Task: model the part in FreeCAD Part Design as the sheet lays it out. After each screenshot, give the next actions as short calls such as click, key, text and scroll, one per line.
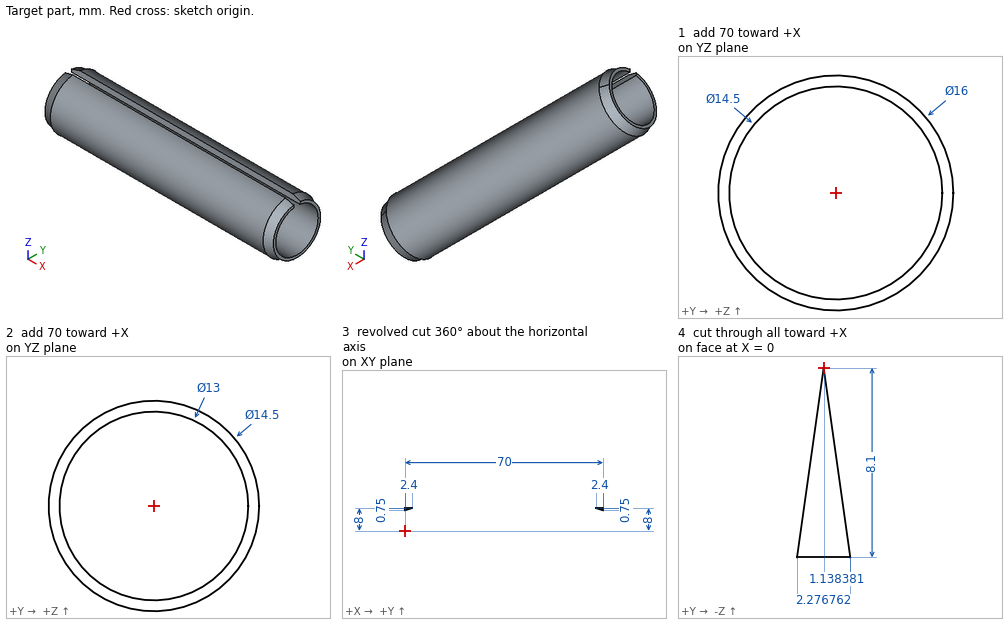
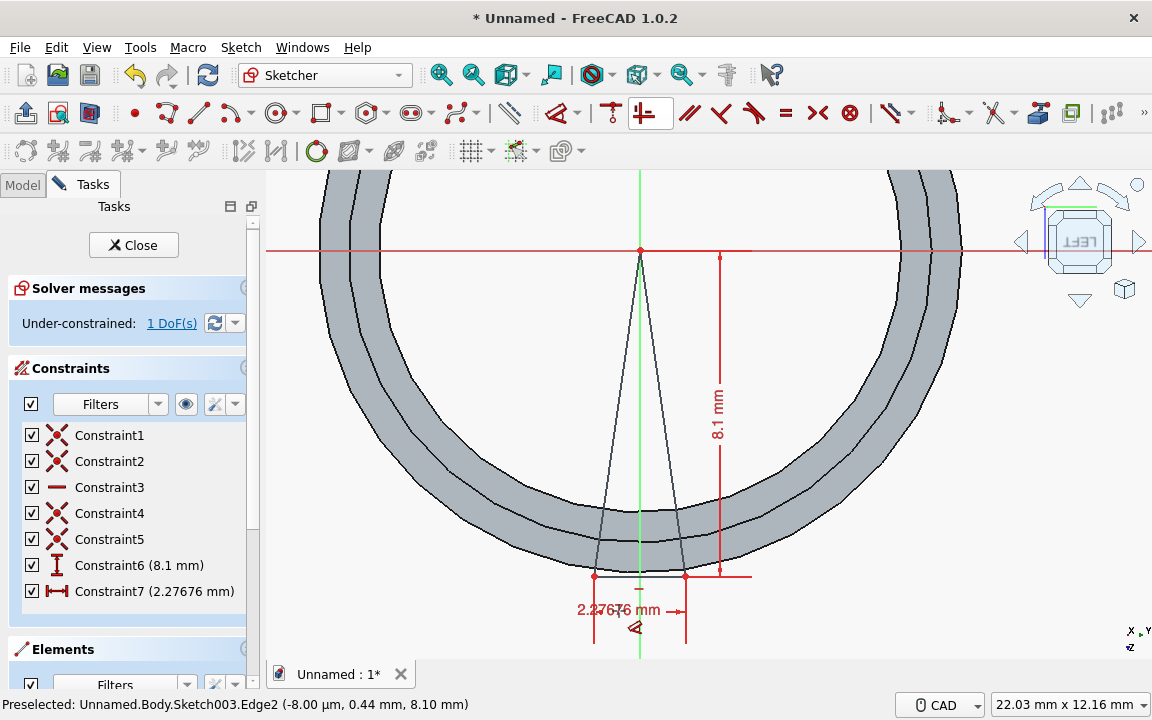
click(686, 577)
click(663, 217)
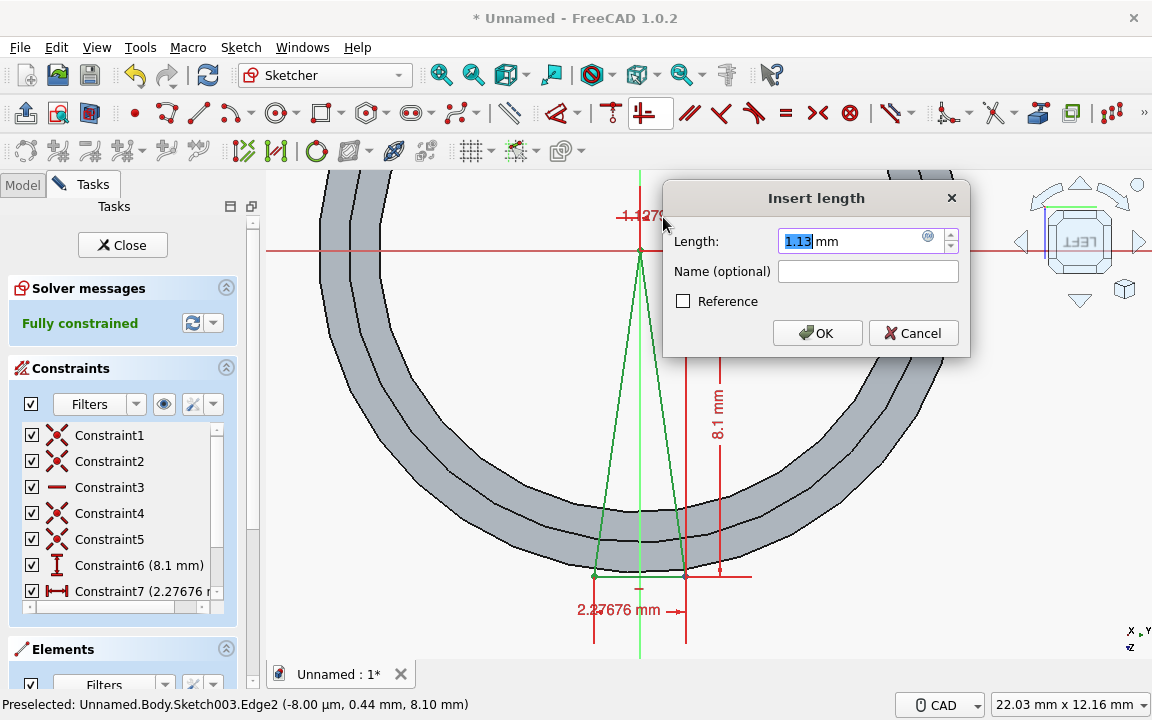
text(1.138381)
key(Return)
key(Escape)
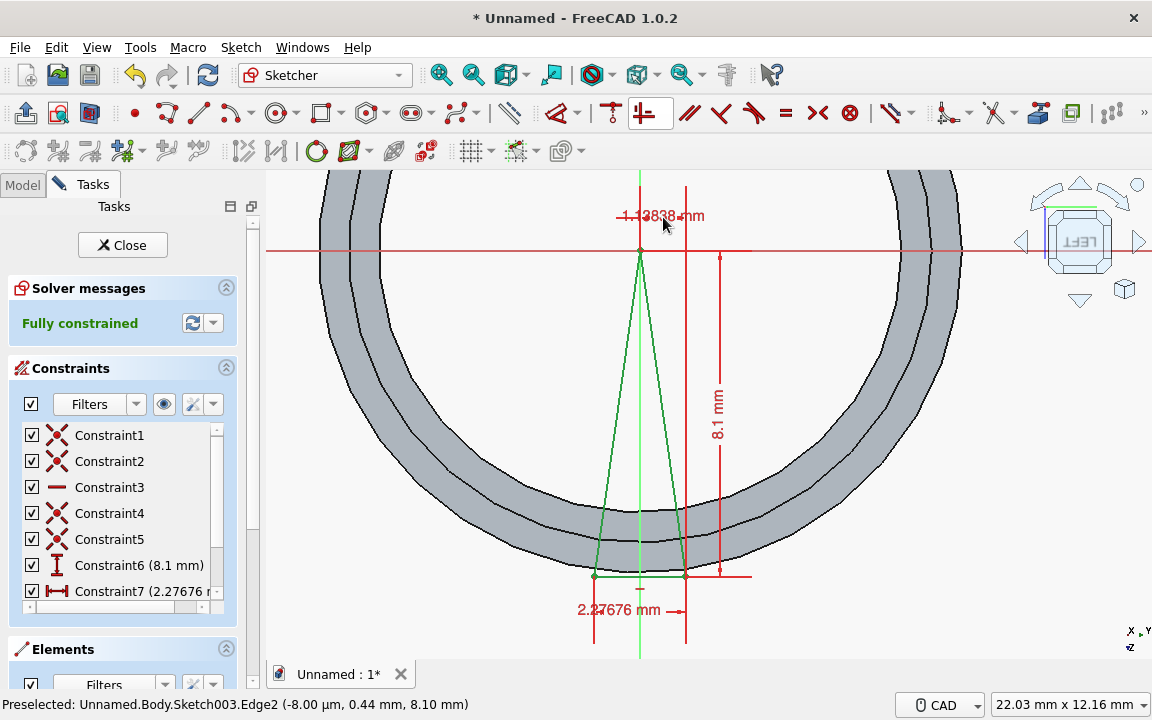
click(123, 245)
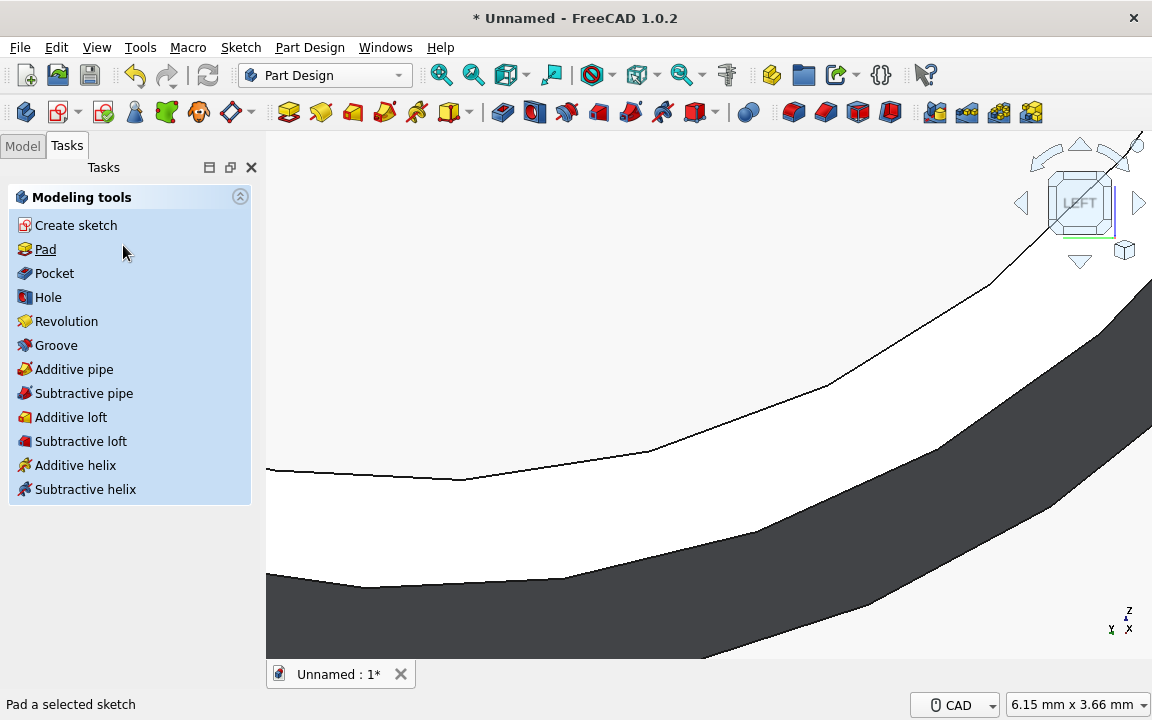
click(504, 112)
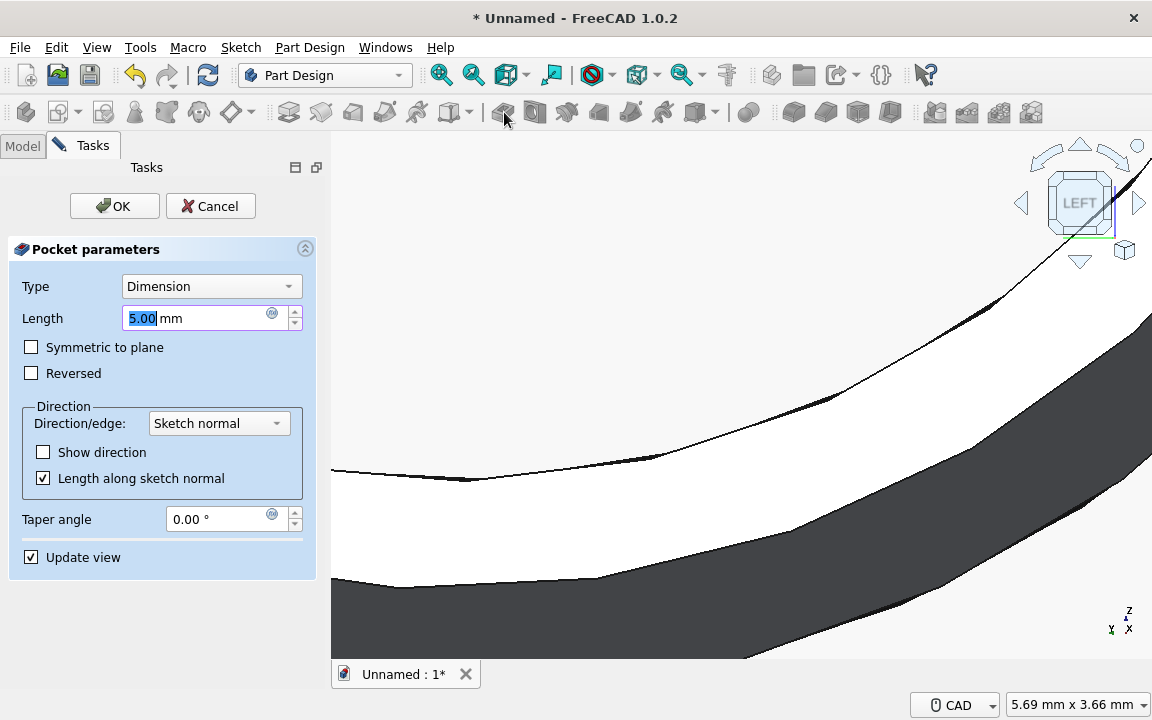
click(212, 286)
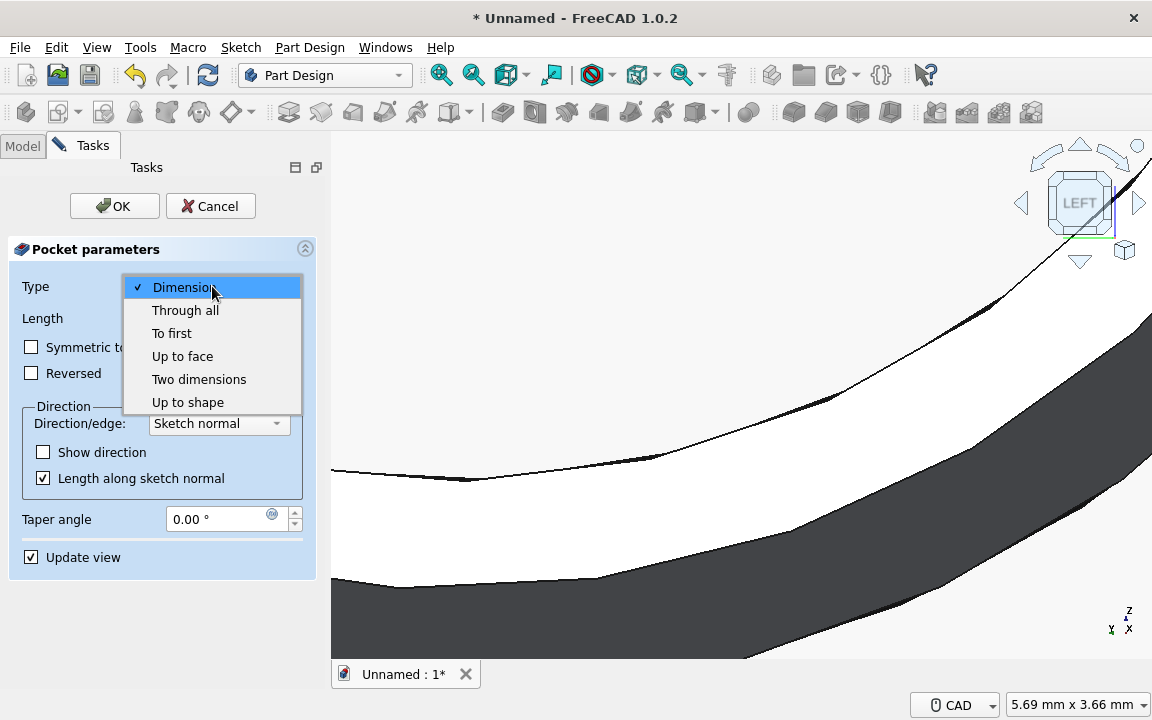
click(212, 310)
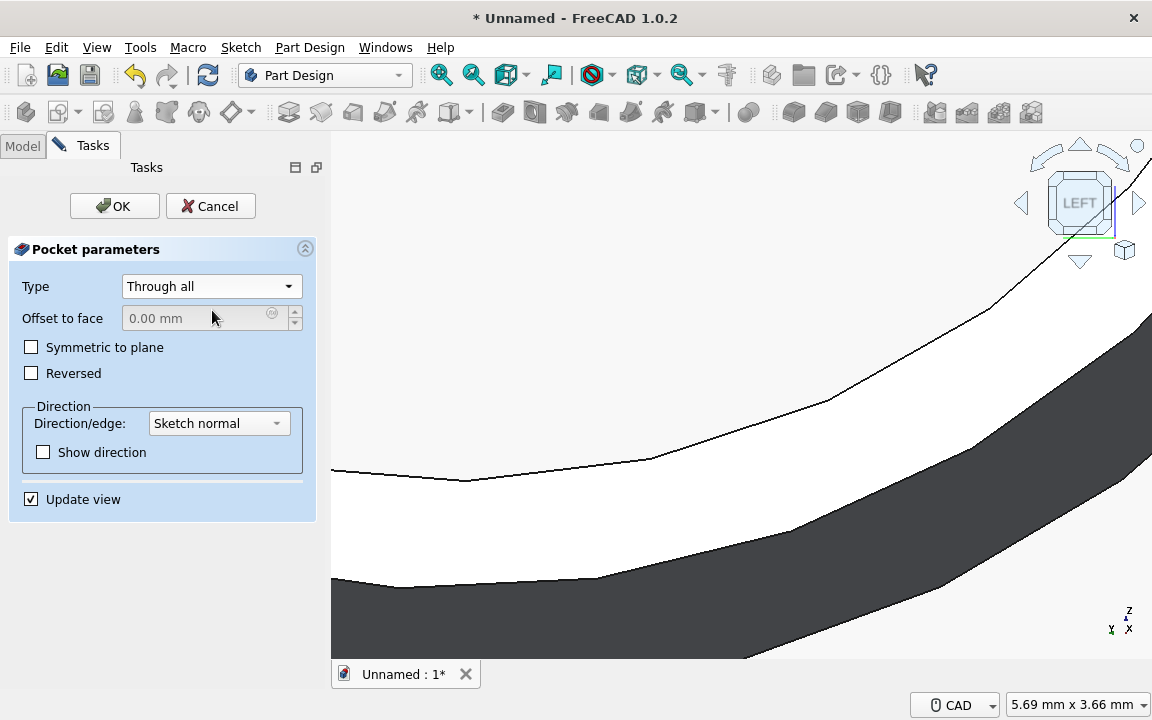
click(115, 206)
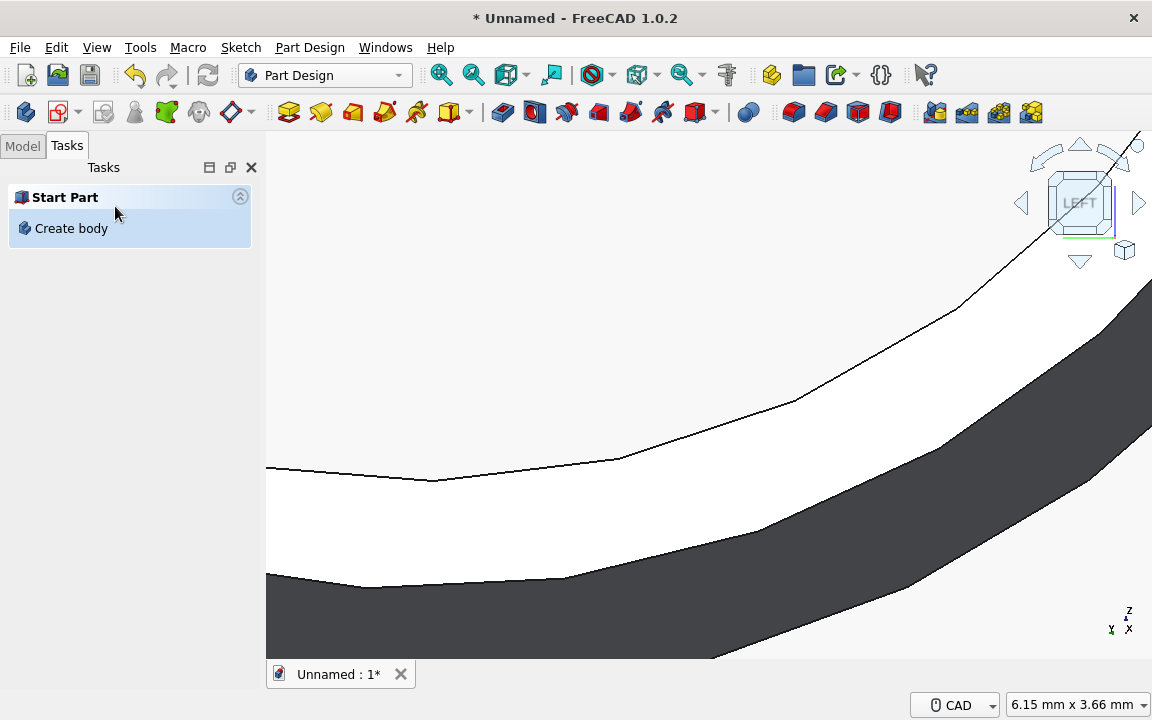
key(0)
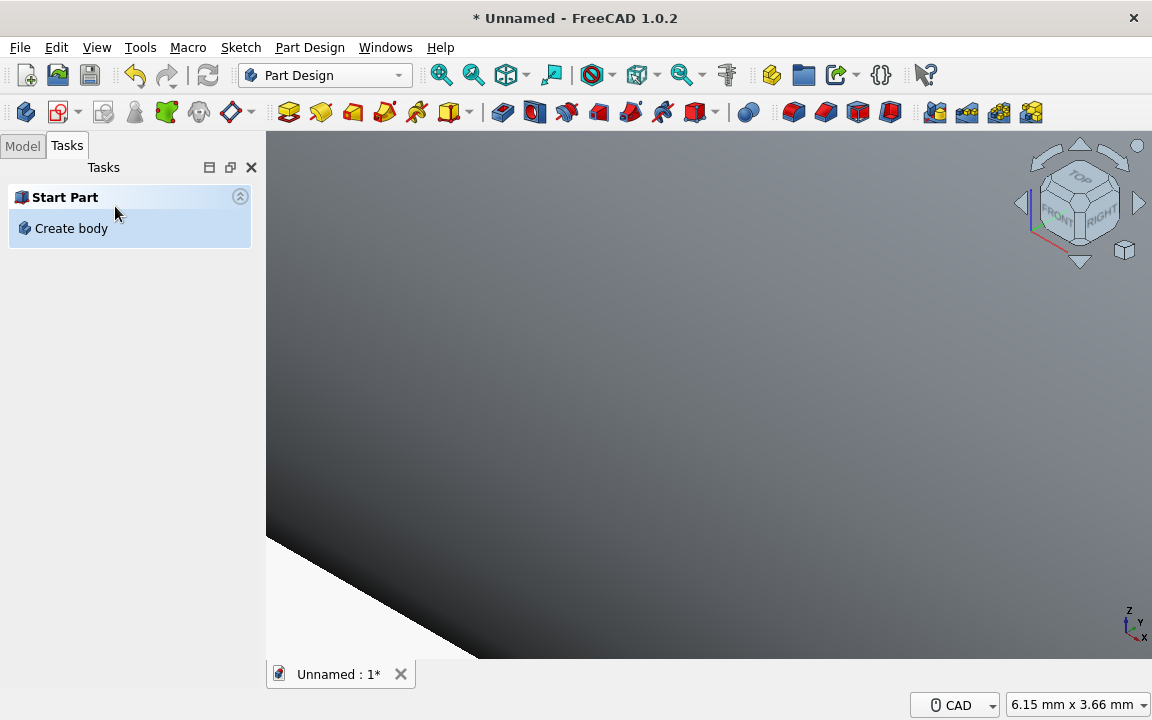
key(v)
key(f)